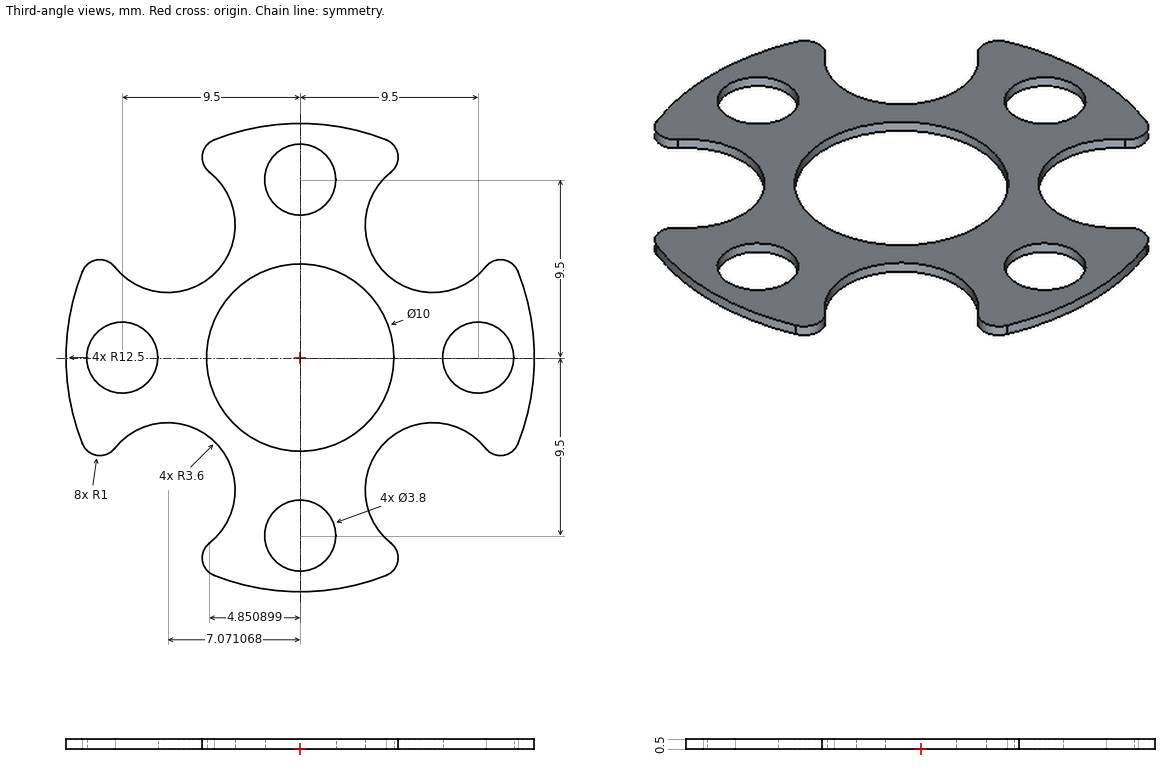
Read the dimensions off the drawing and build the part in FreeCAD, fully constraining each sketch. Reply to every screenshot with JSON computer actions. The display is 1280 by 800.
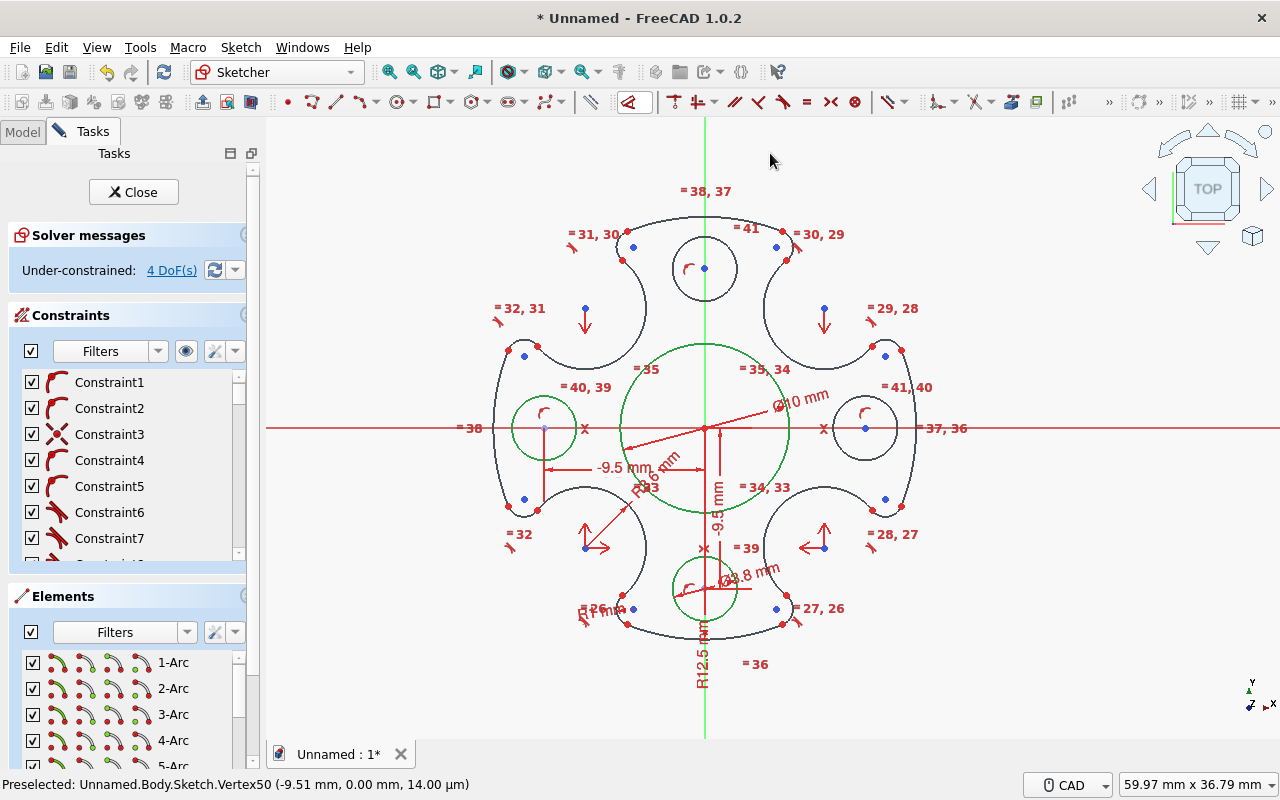
{"action": "left_click", "coordinate": [865, 428]}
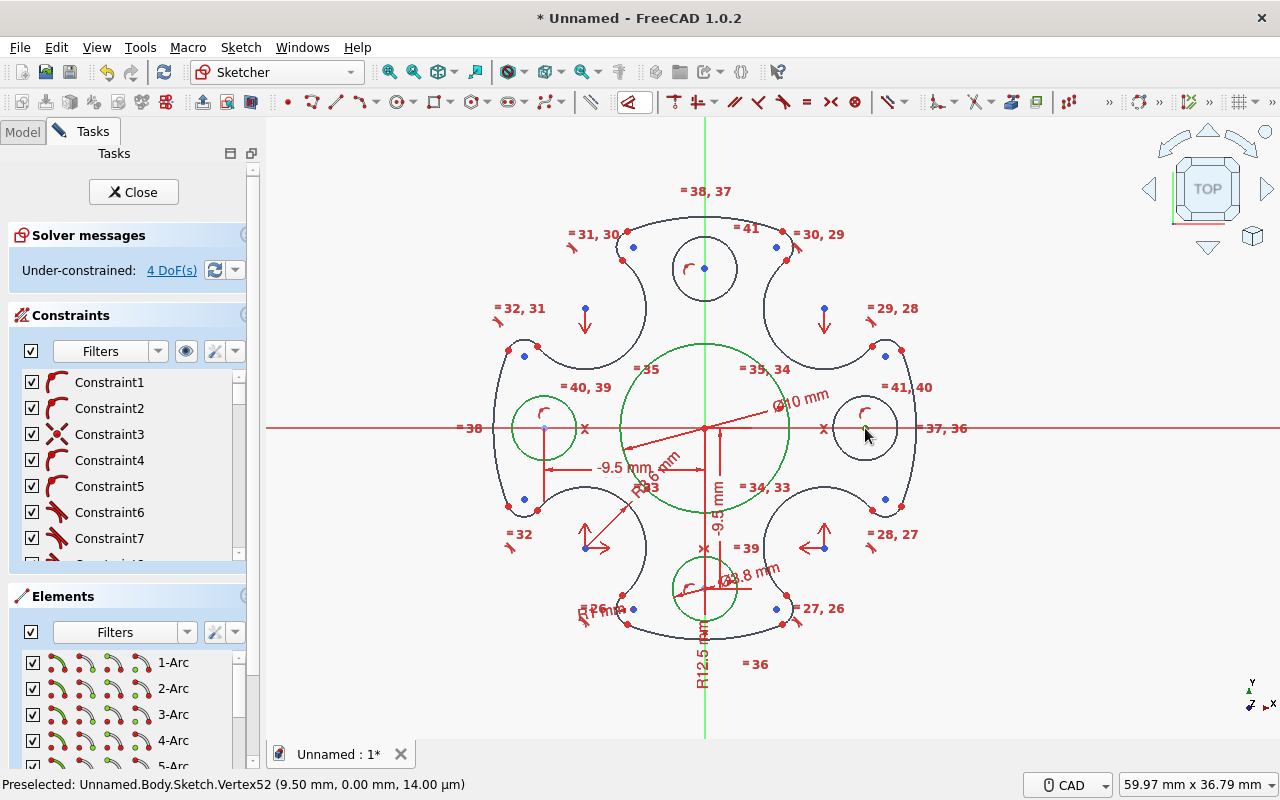
{"action": "key", "text": "l"}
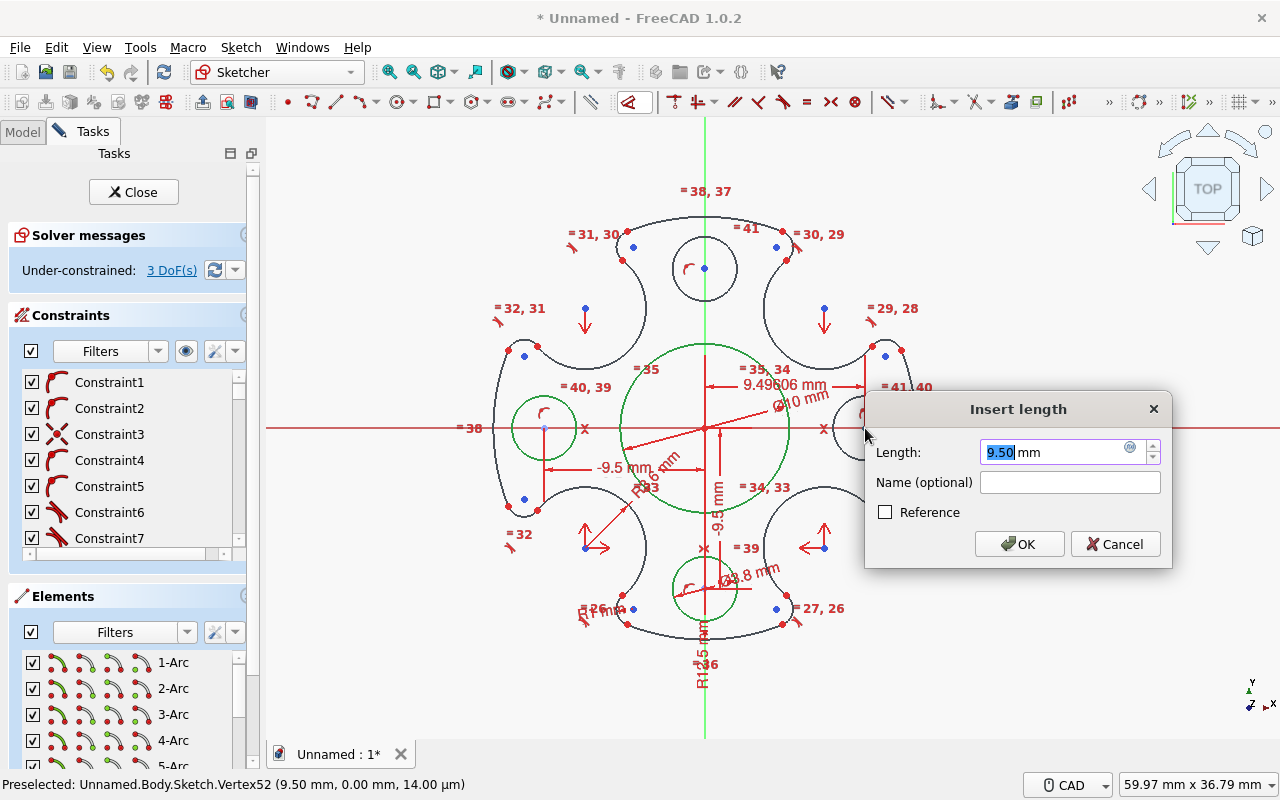
{"action": "type", "text": "9.5"}
{"action": "key", "text": "Return"}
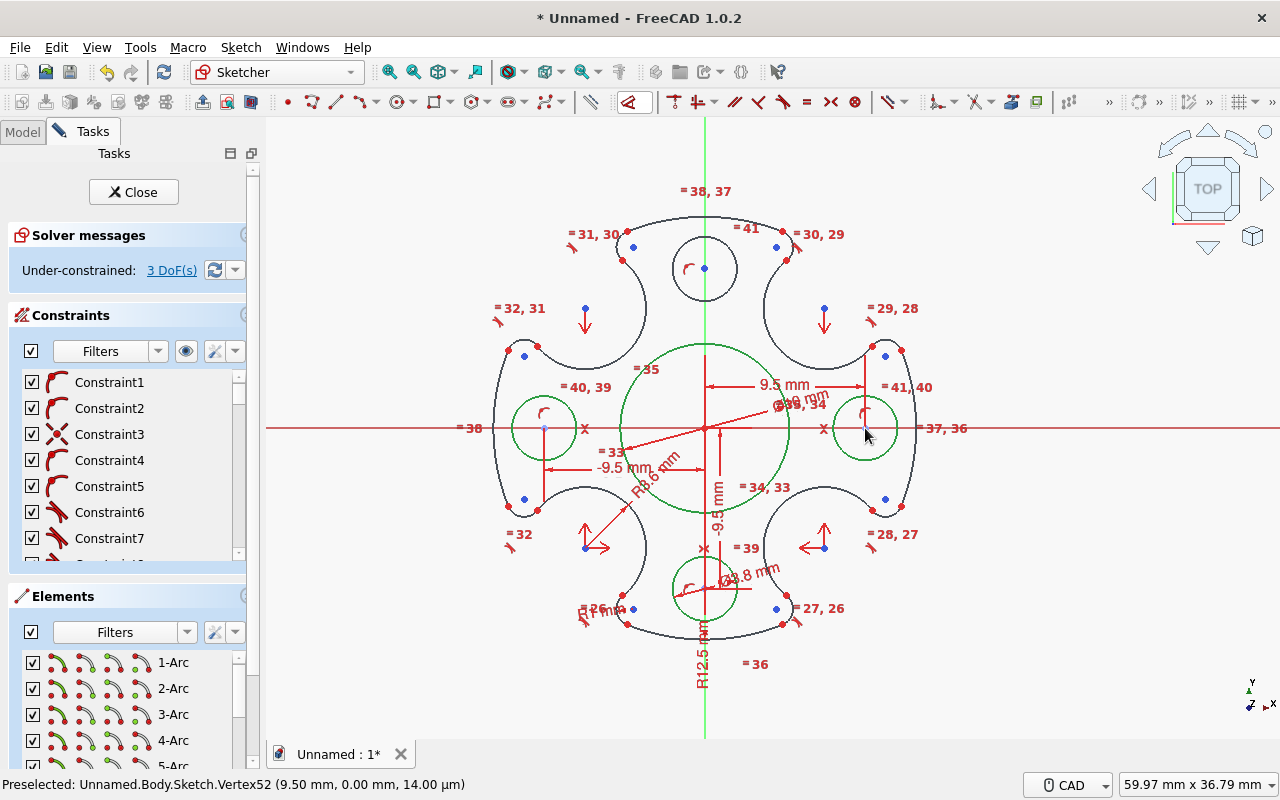
{"action": "left_click", "coordinate": [705, 269]}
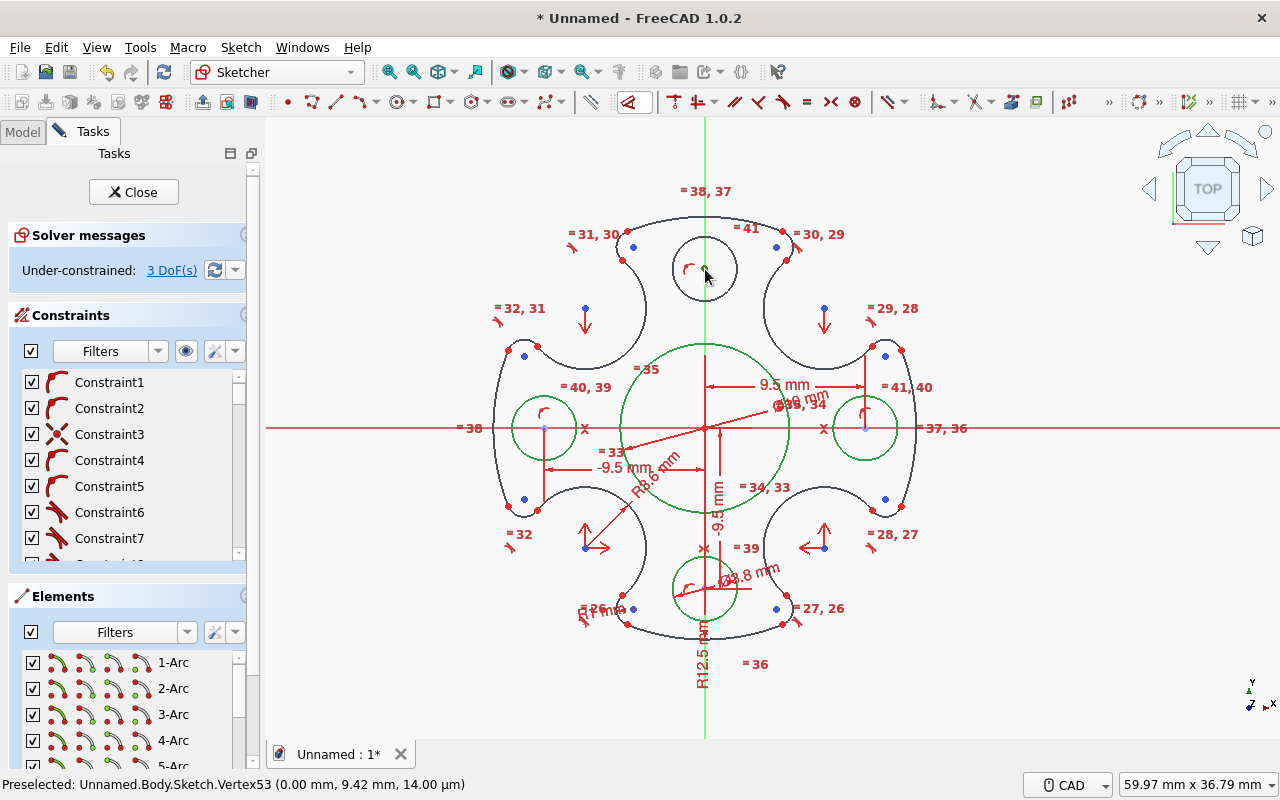
{"action": "key", "text": "i"}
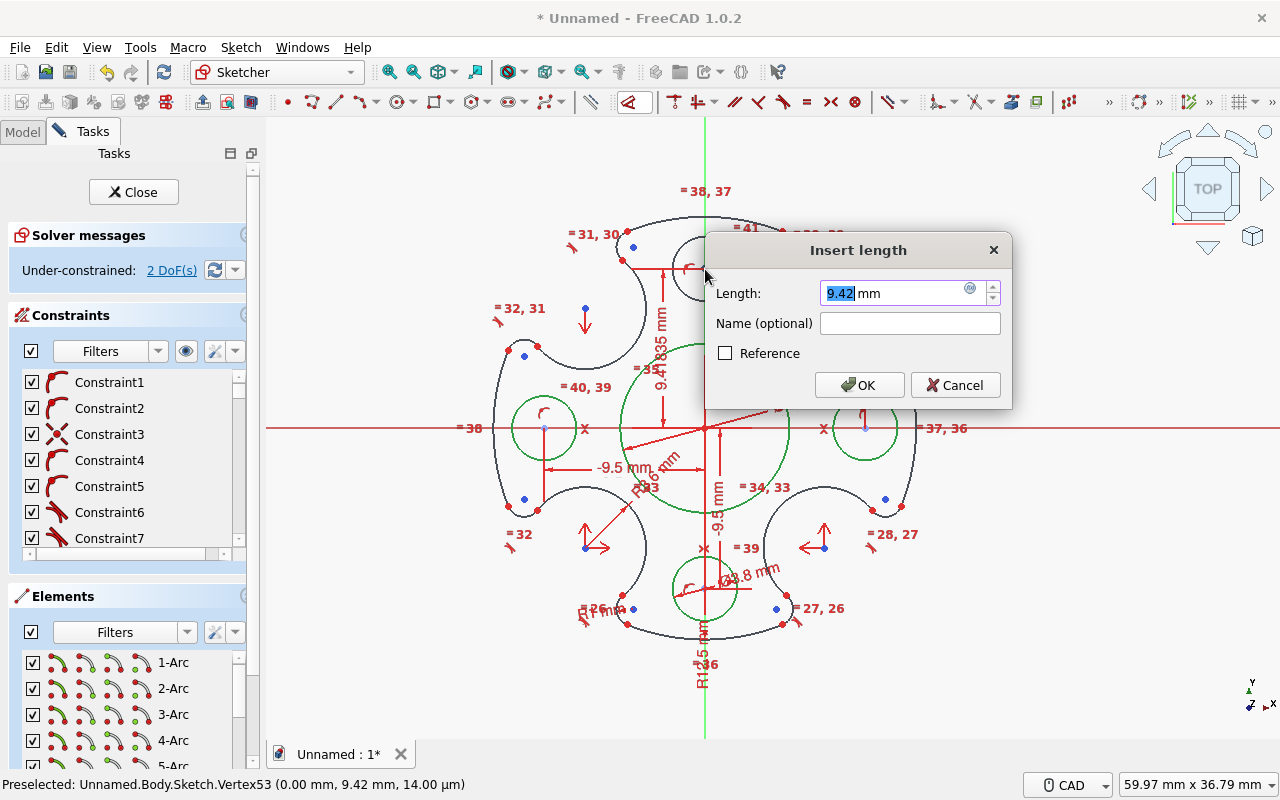
{"action": "type", "text": "9.5"}
{"action": "key", "text": "Return"}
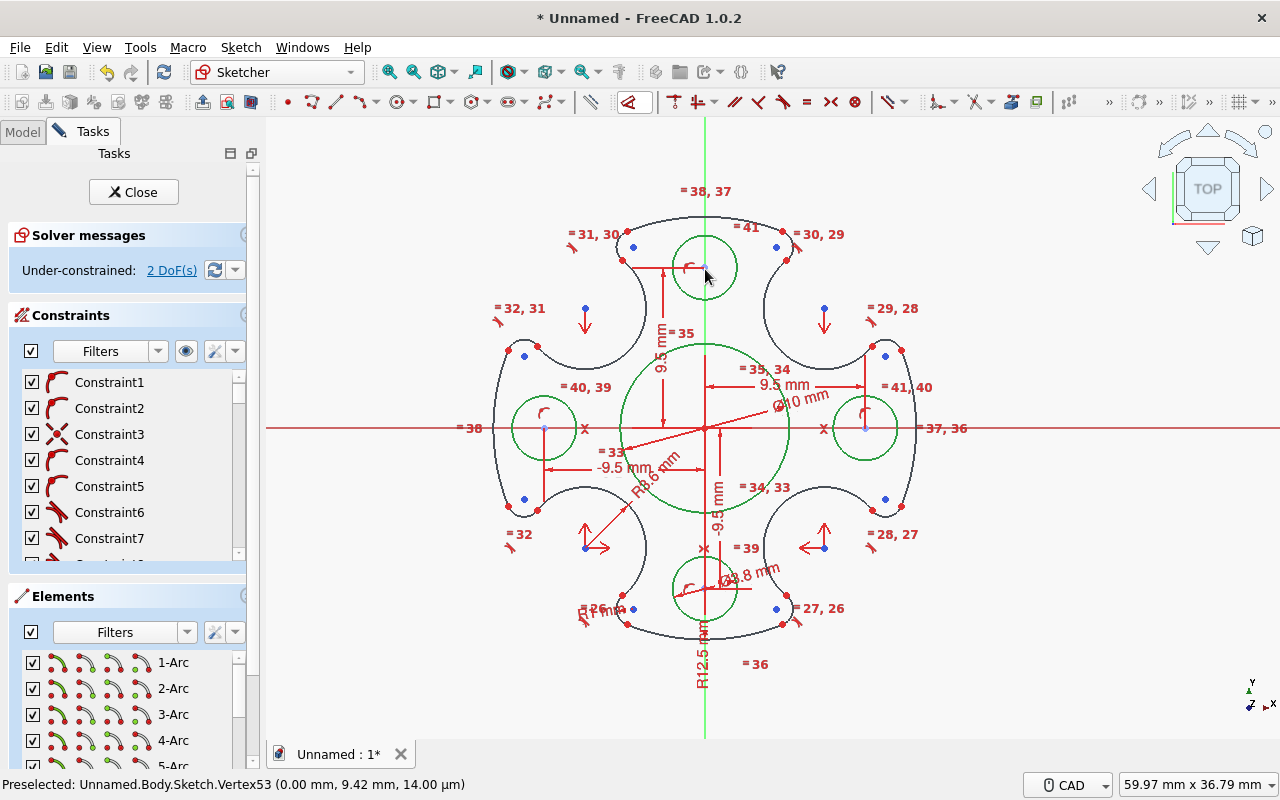
{"action": "left_click", "coordinate": [623, 596]}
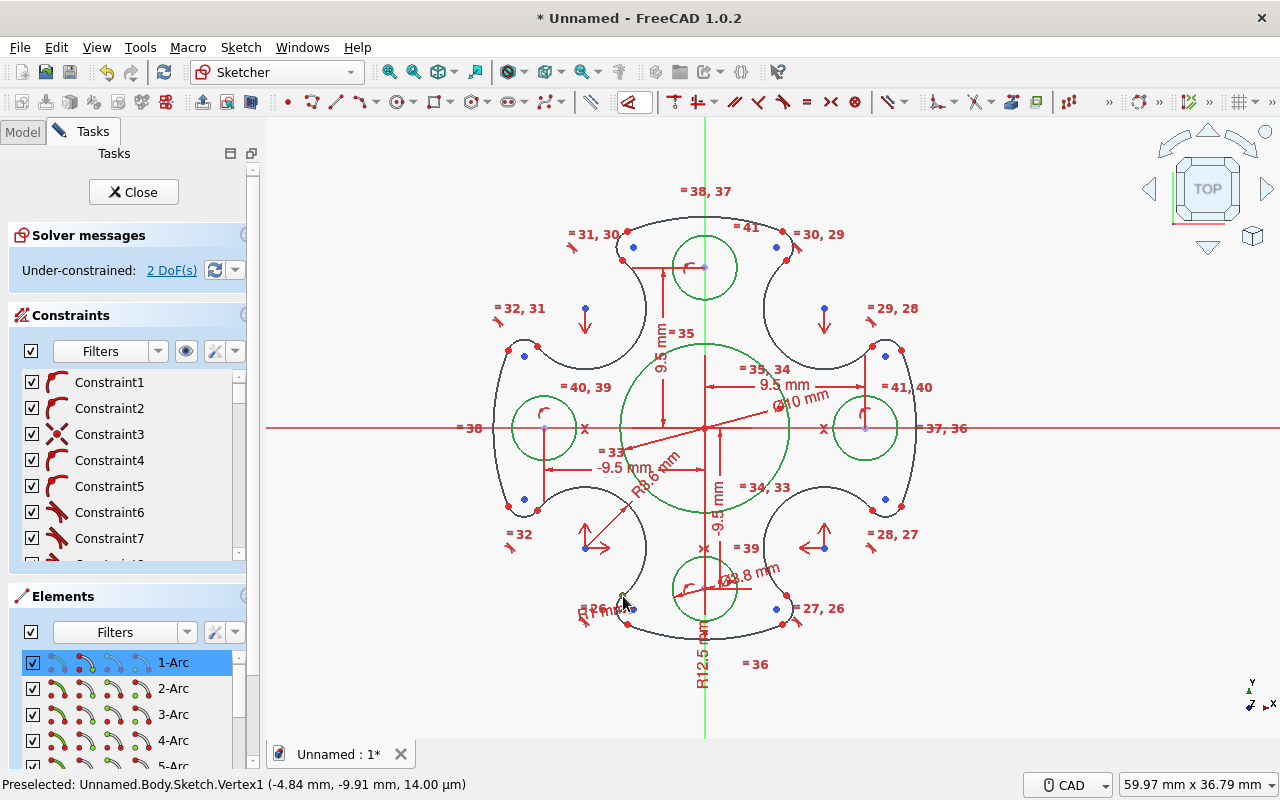
{"action": "left_click", "coordinate": [646, 102]}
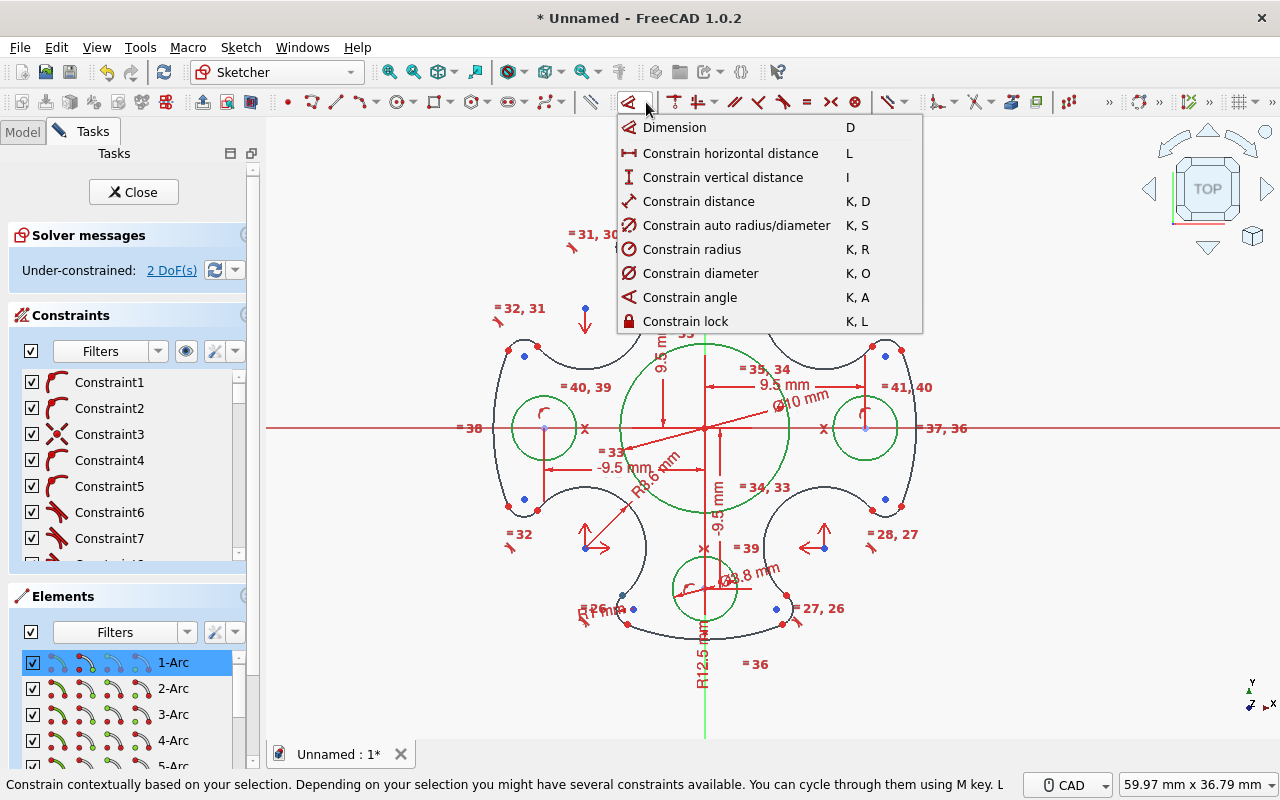
{"action": "left_click", "coordinate": [770, 153]}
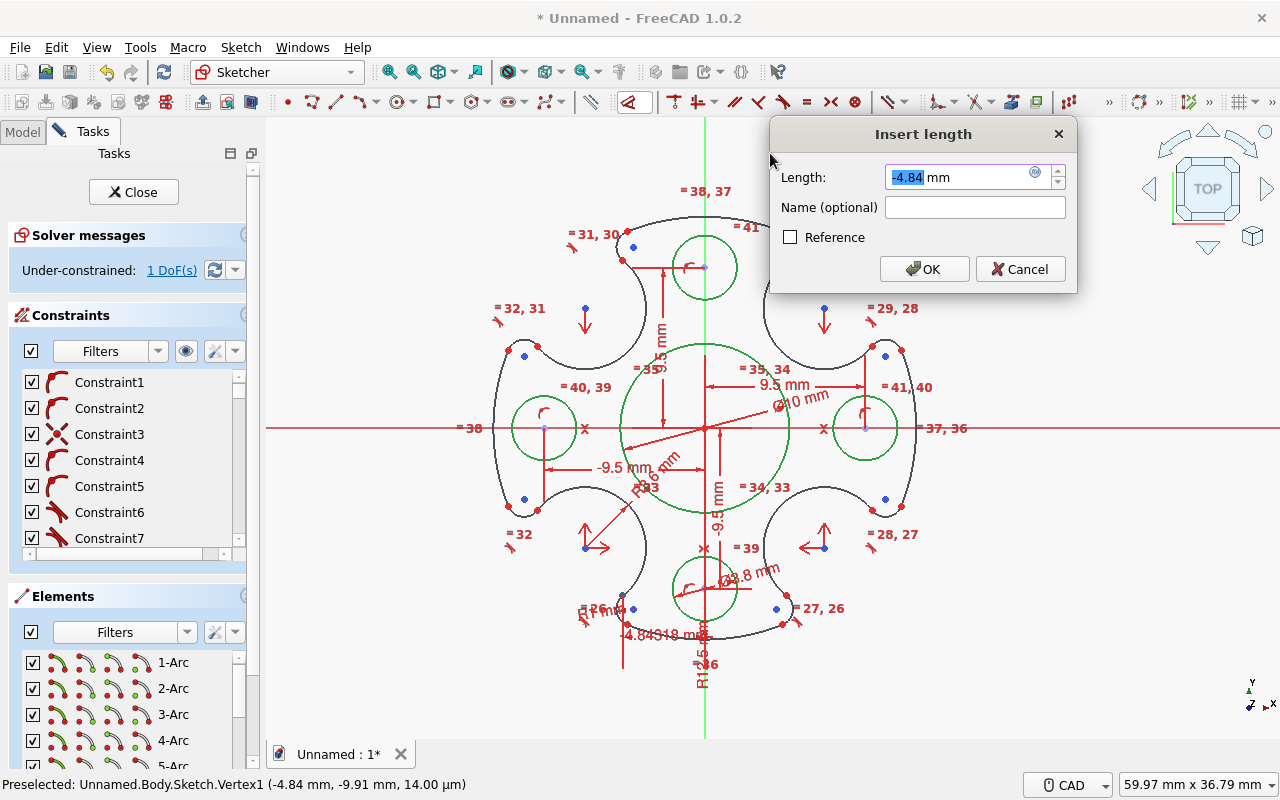
{"action": "type", "text": "-4.850899"}
{"action": "key", "text": "Return"}